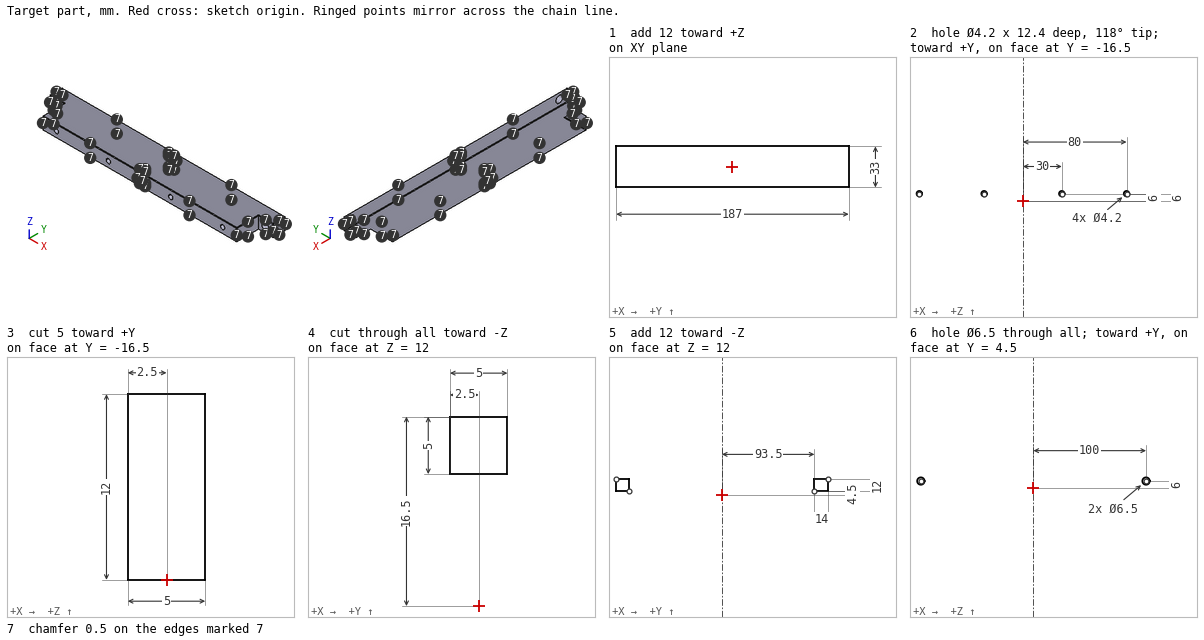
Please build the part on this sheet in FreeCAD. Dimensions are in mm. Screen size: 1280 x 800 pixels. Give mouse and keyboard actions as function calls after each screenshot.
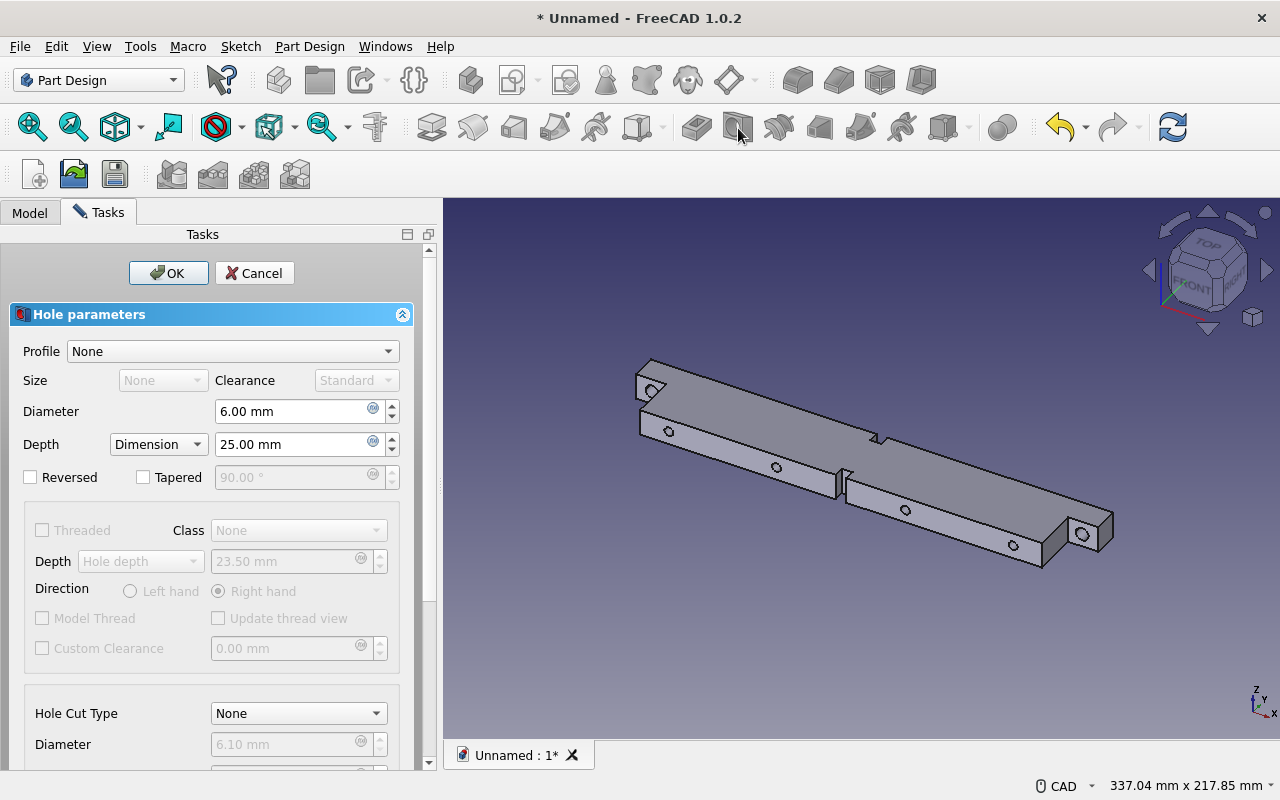
triple_click(300, 412)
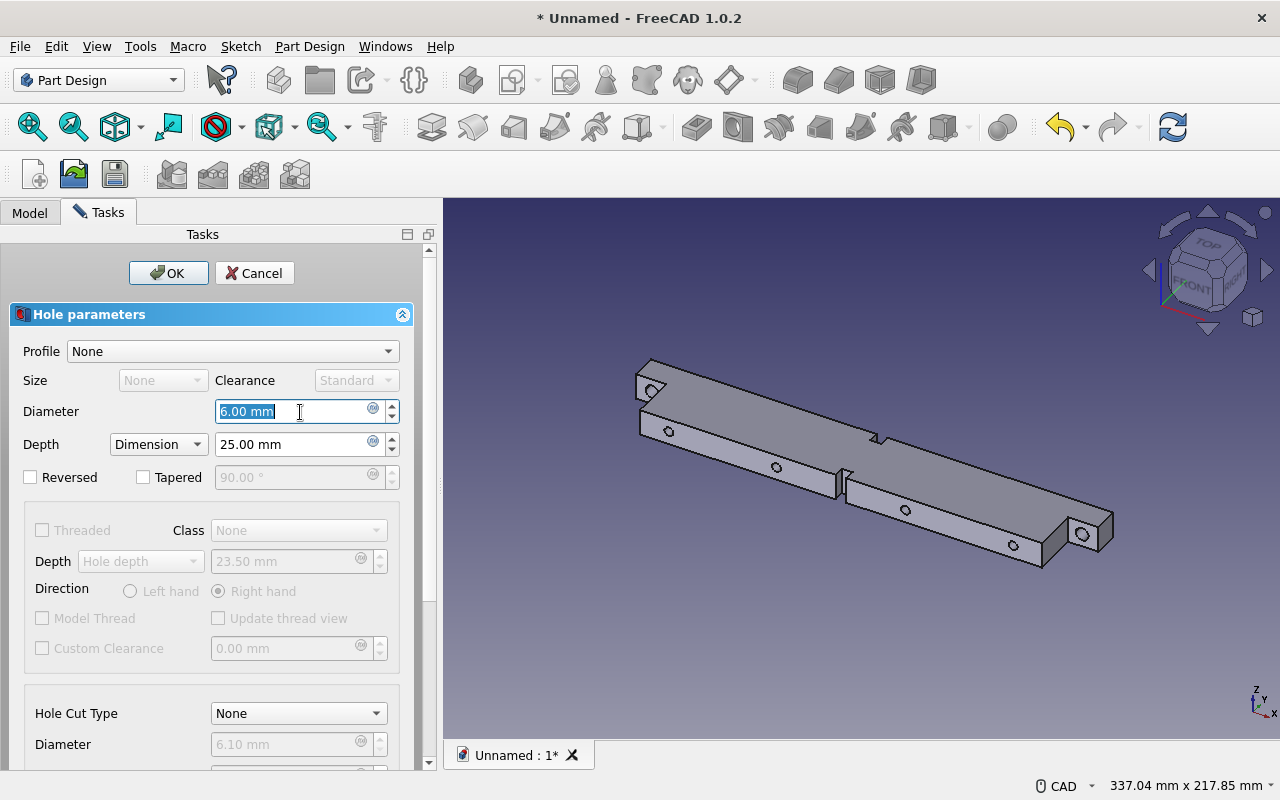
text(6.5)
key(Tab)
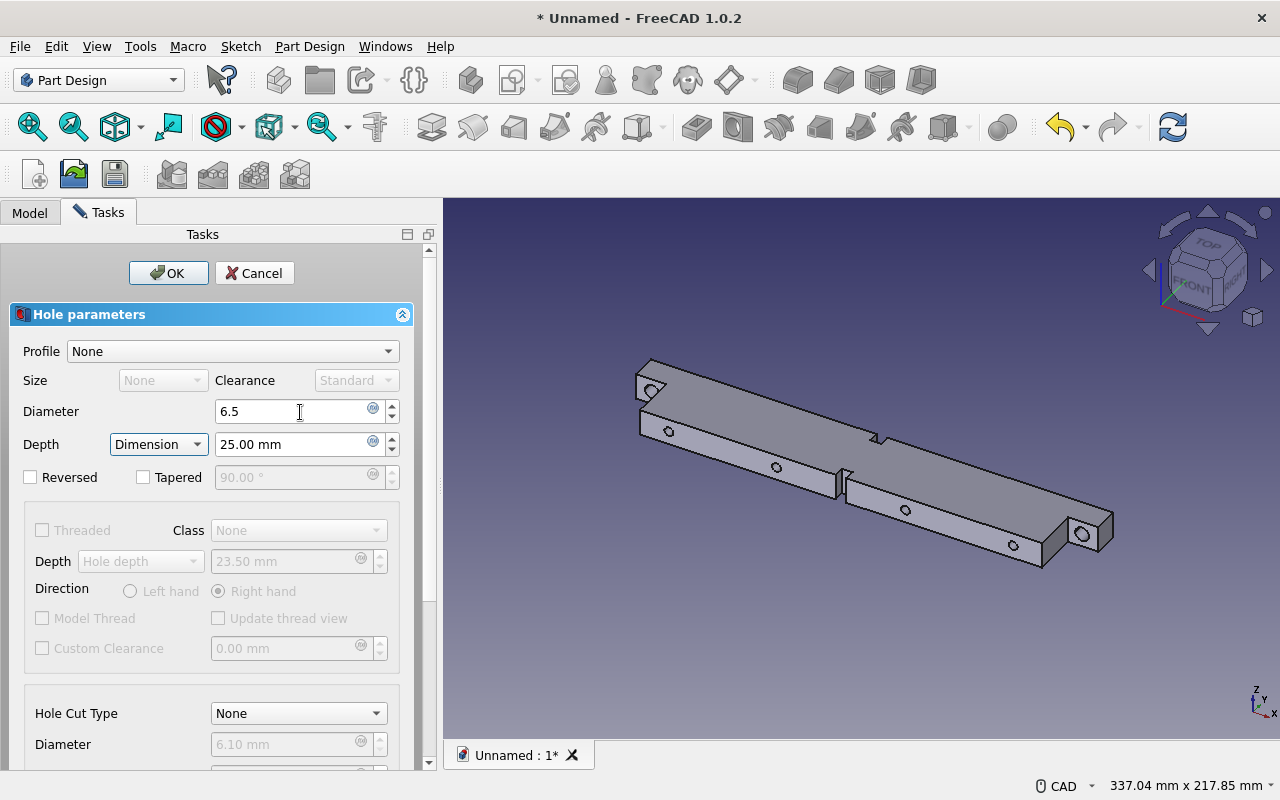
click(160, 444)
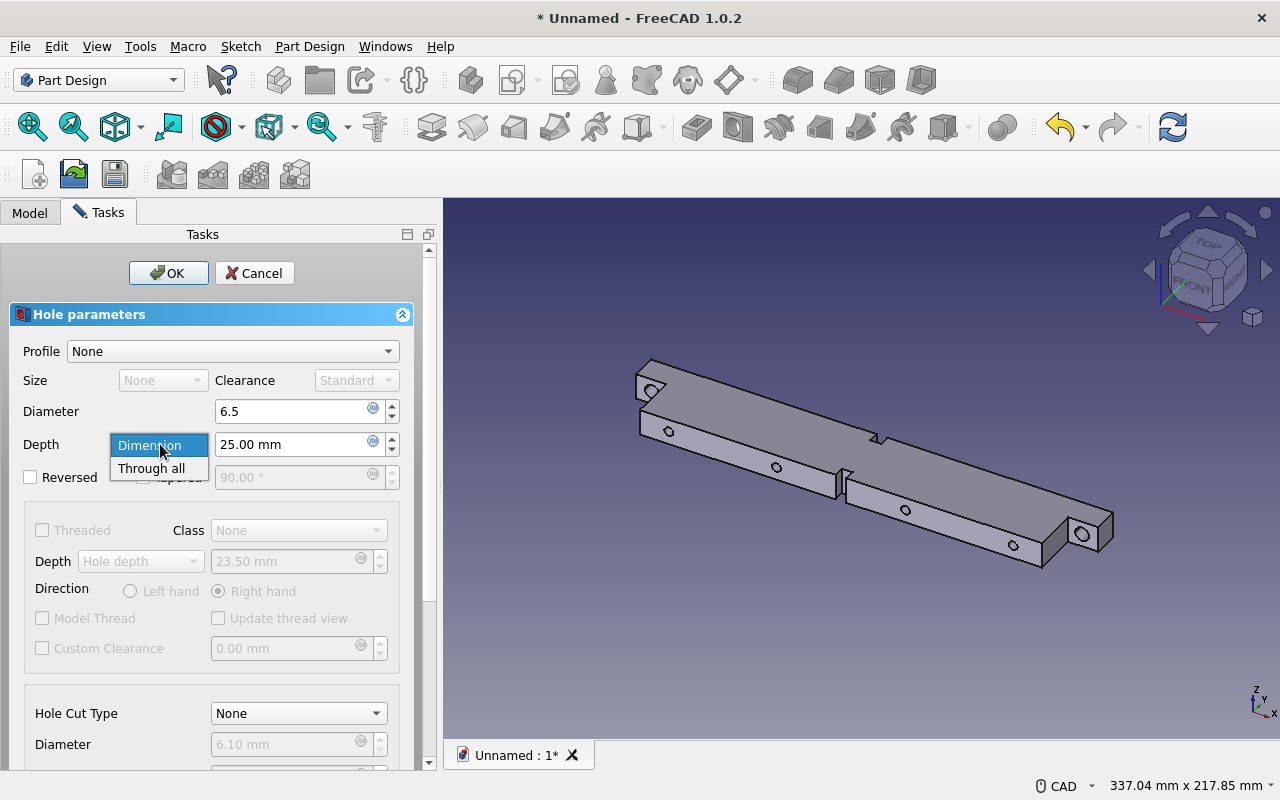
click(158, 468)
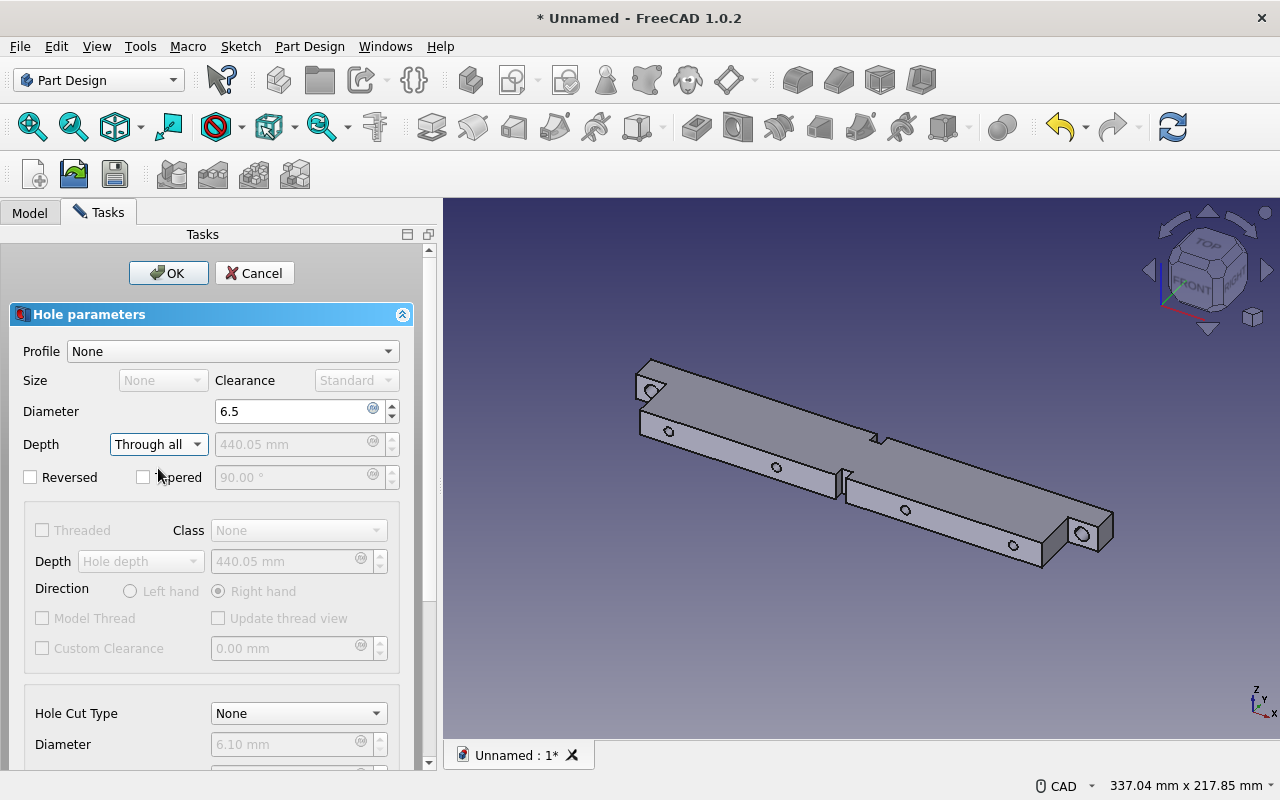
click(169, 273)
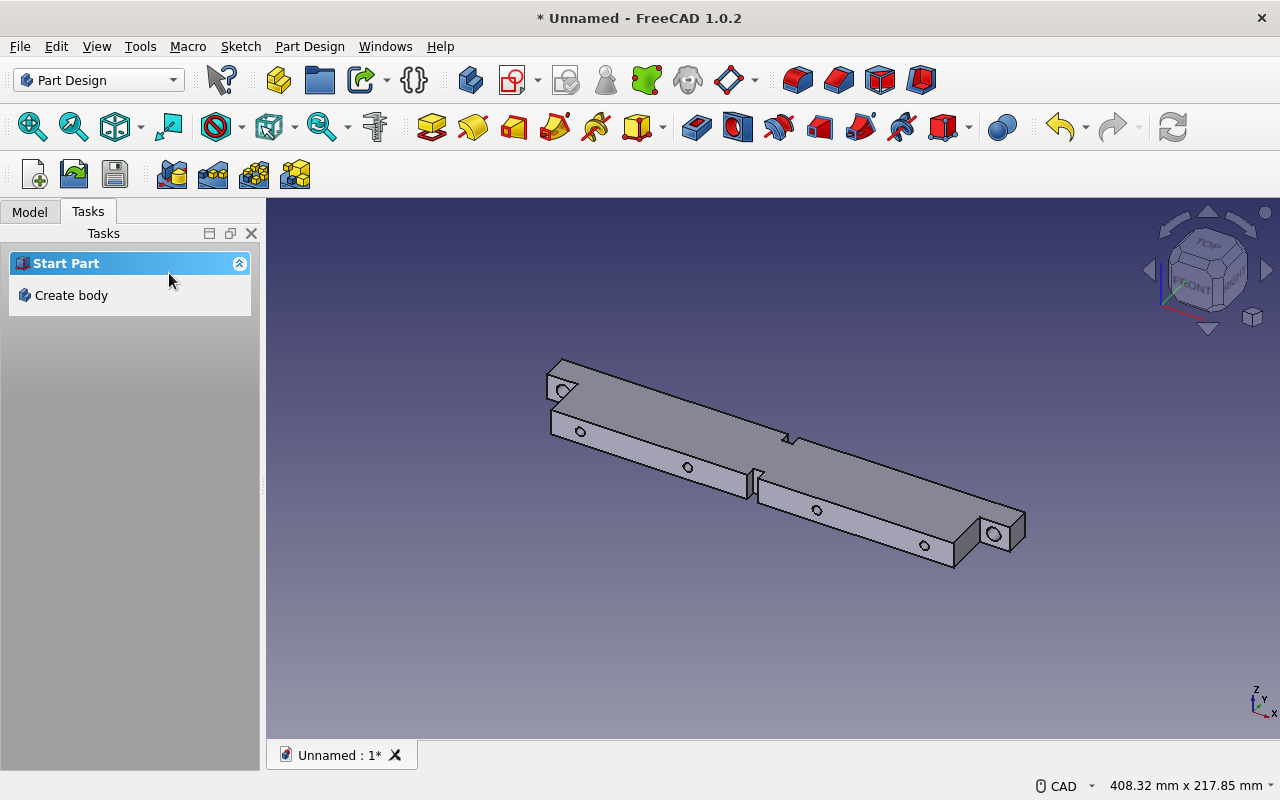
click(905, 499)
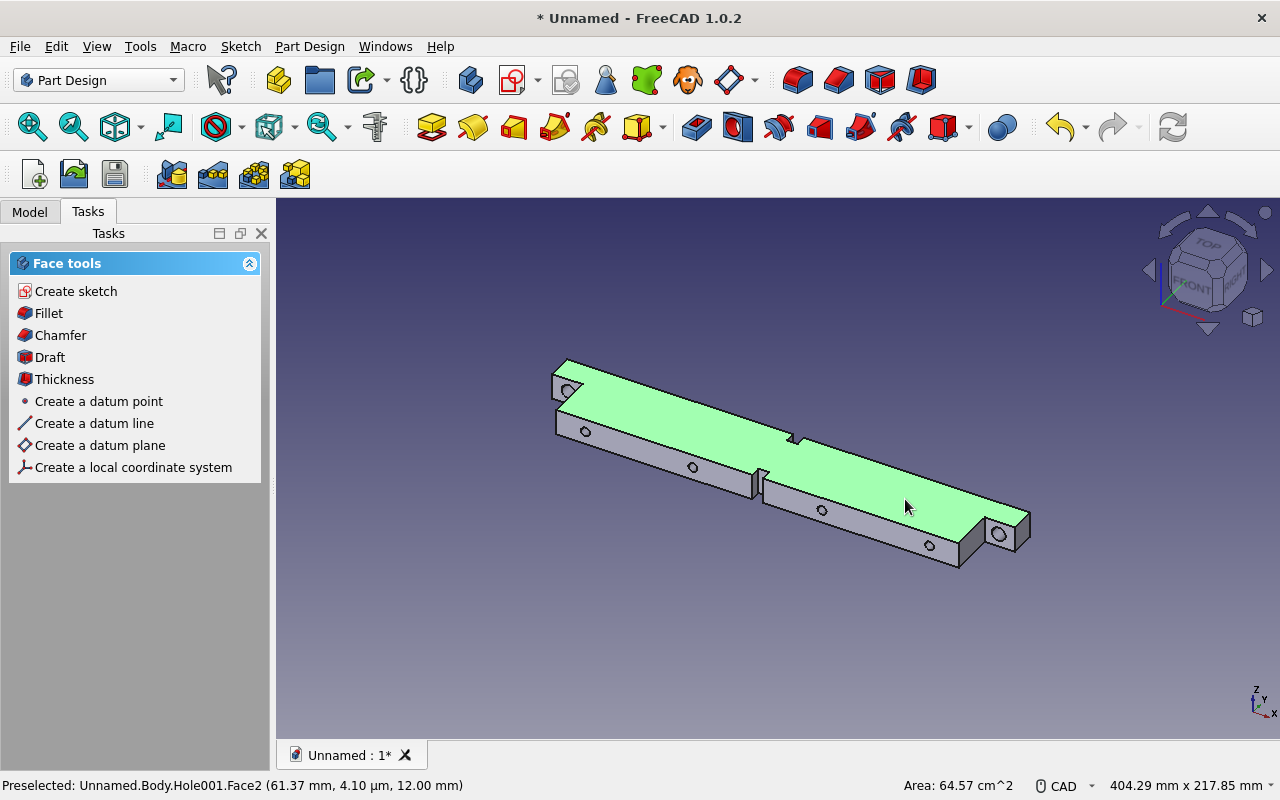
click(752, 486, ctrl)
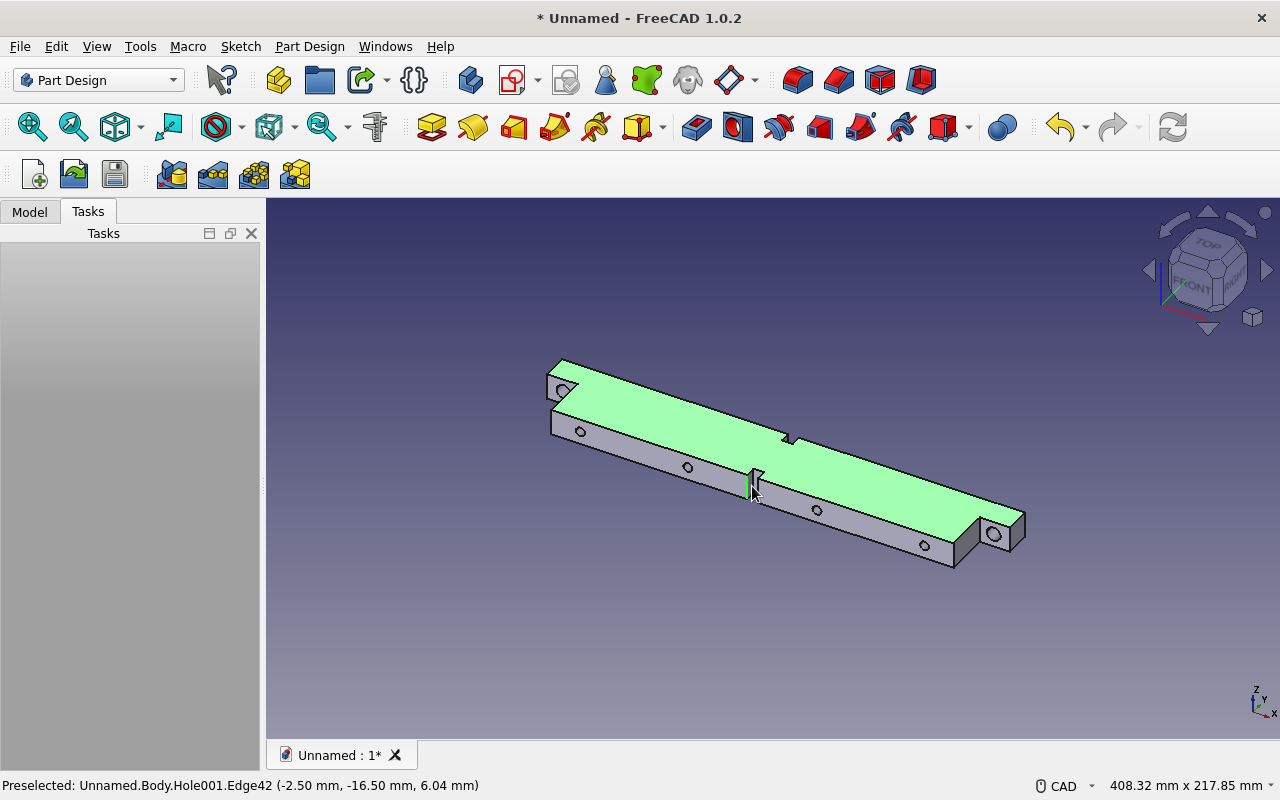
click(1010, 539, ctrl)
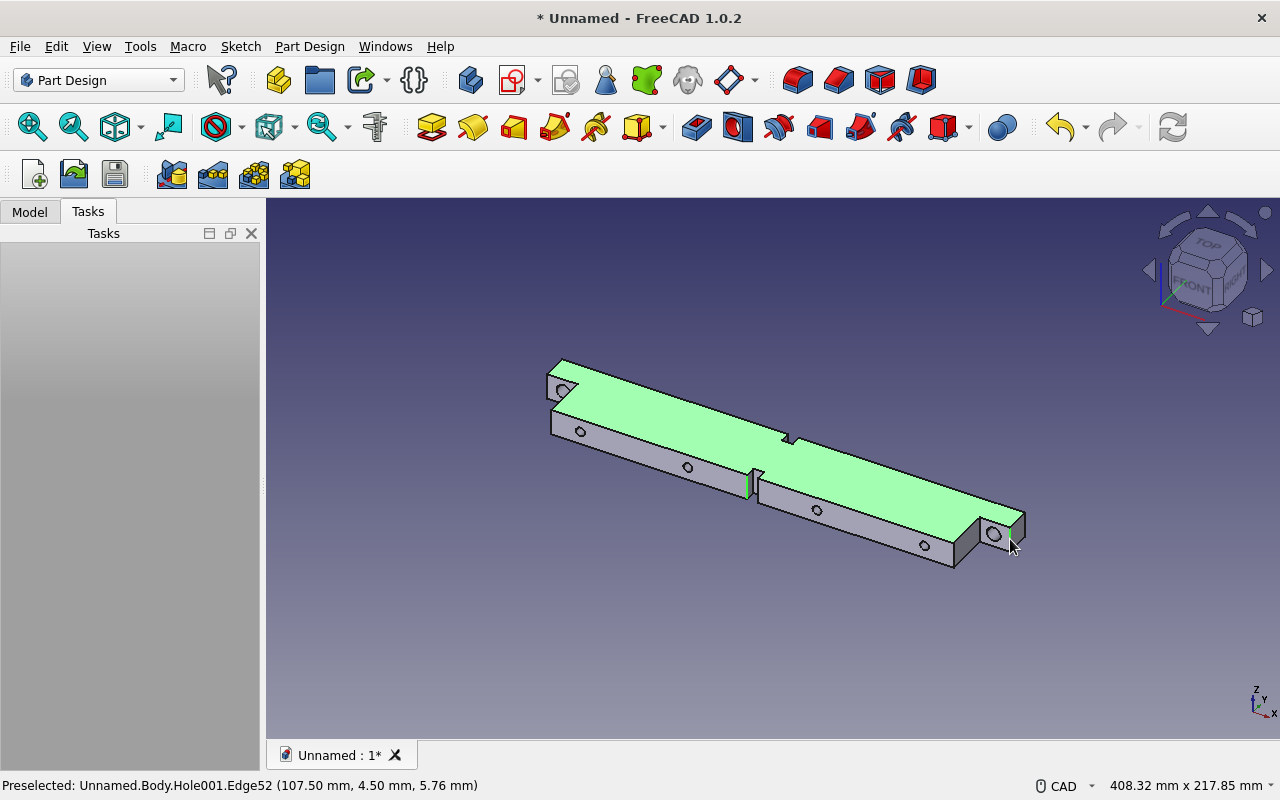
click(954, 554, ctrl)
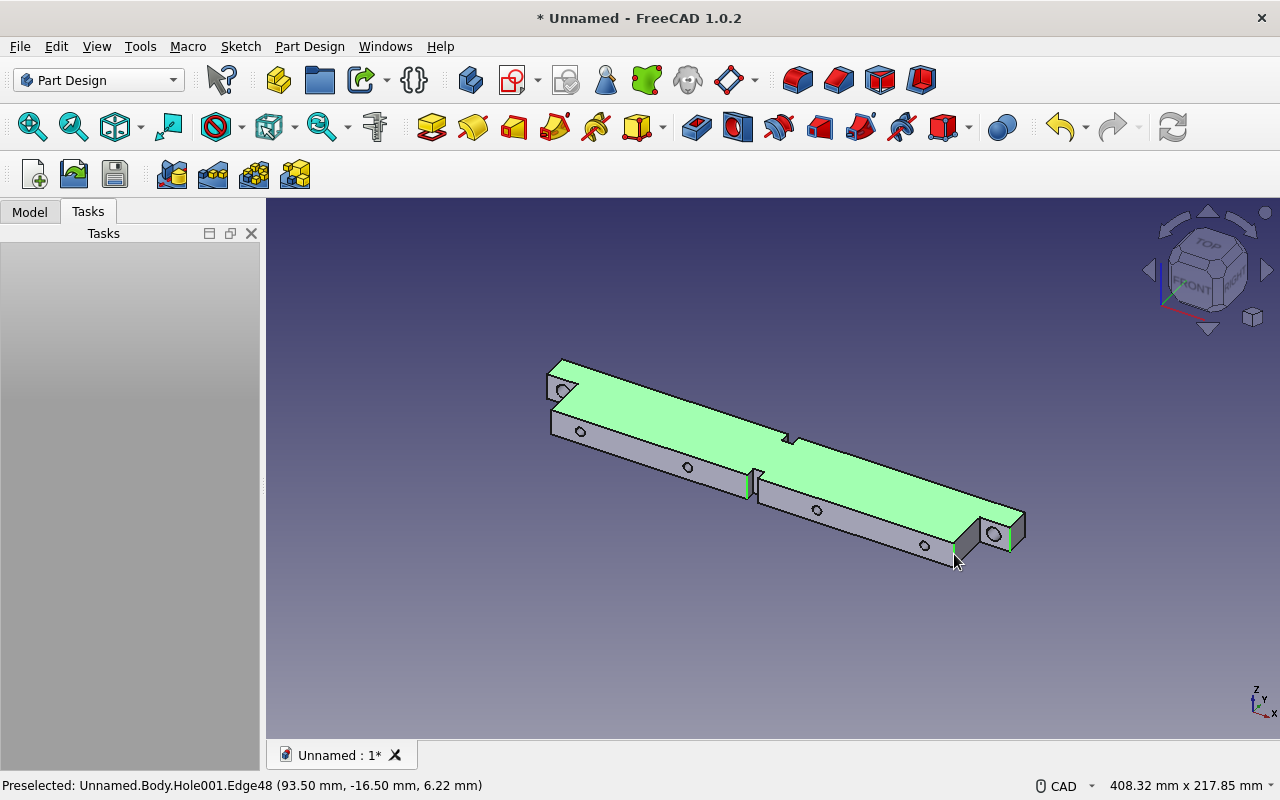
key(0)